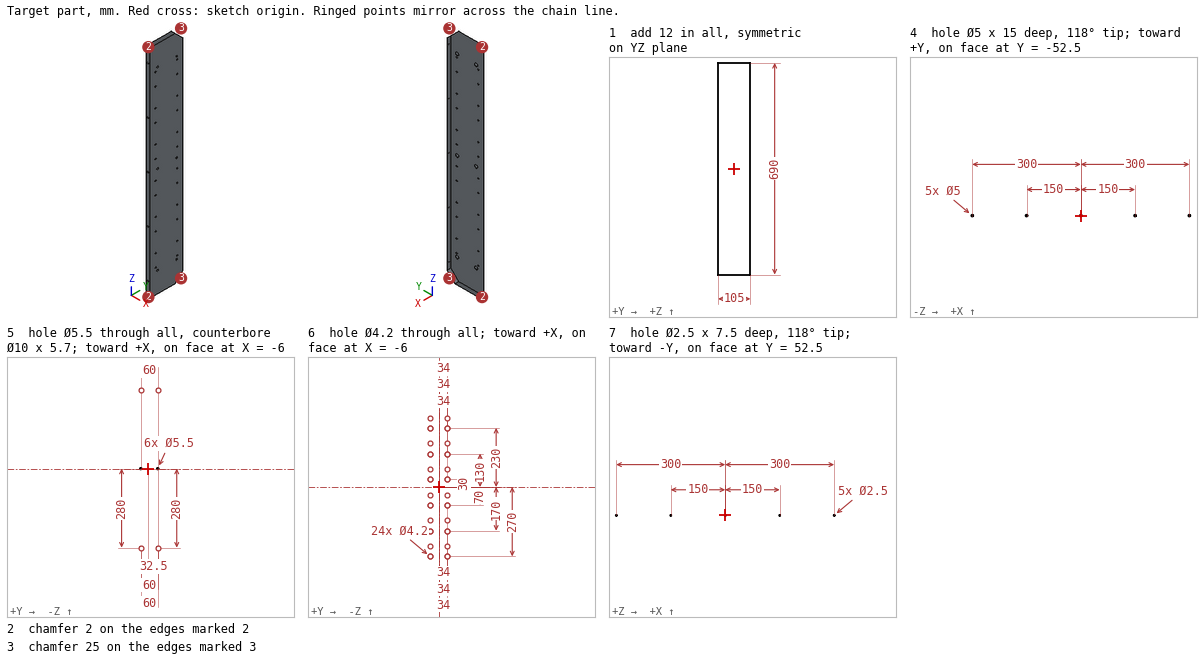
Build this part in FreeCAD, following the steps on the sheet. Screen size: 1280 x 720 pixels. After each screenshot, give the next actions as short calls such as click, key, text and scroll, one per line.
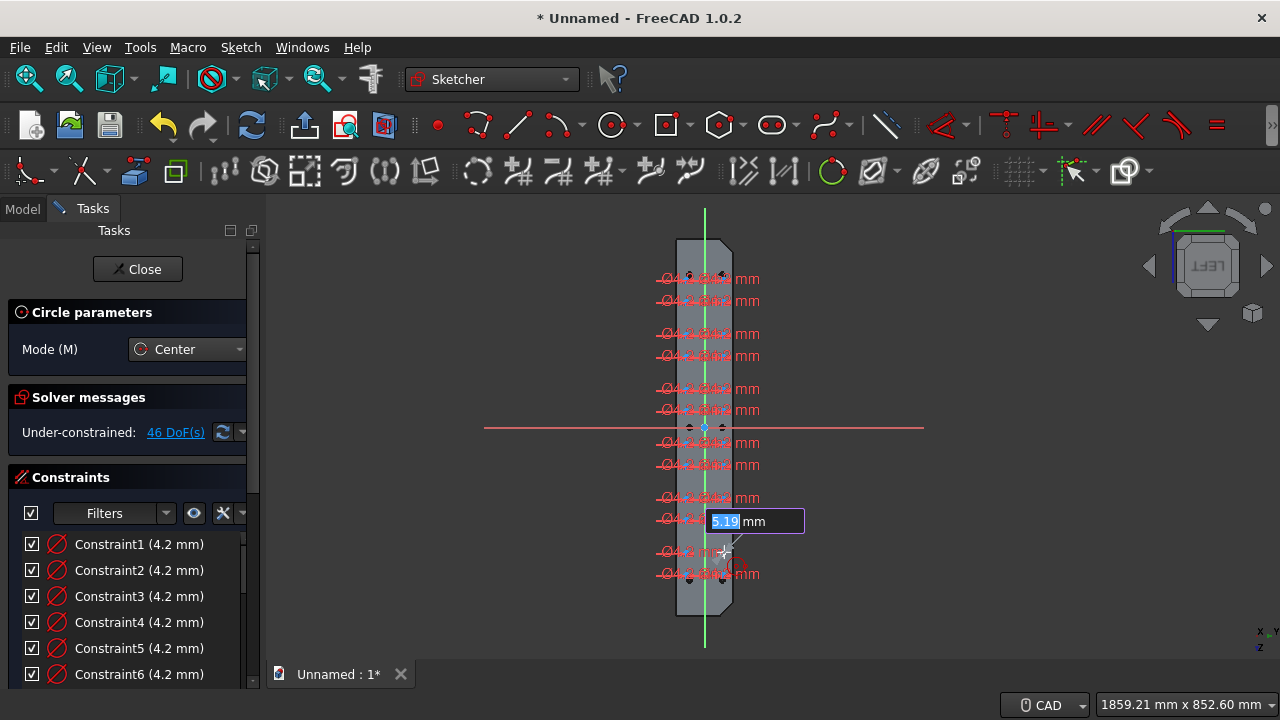
text(4.2)
key(Return)
key(Escape)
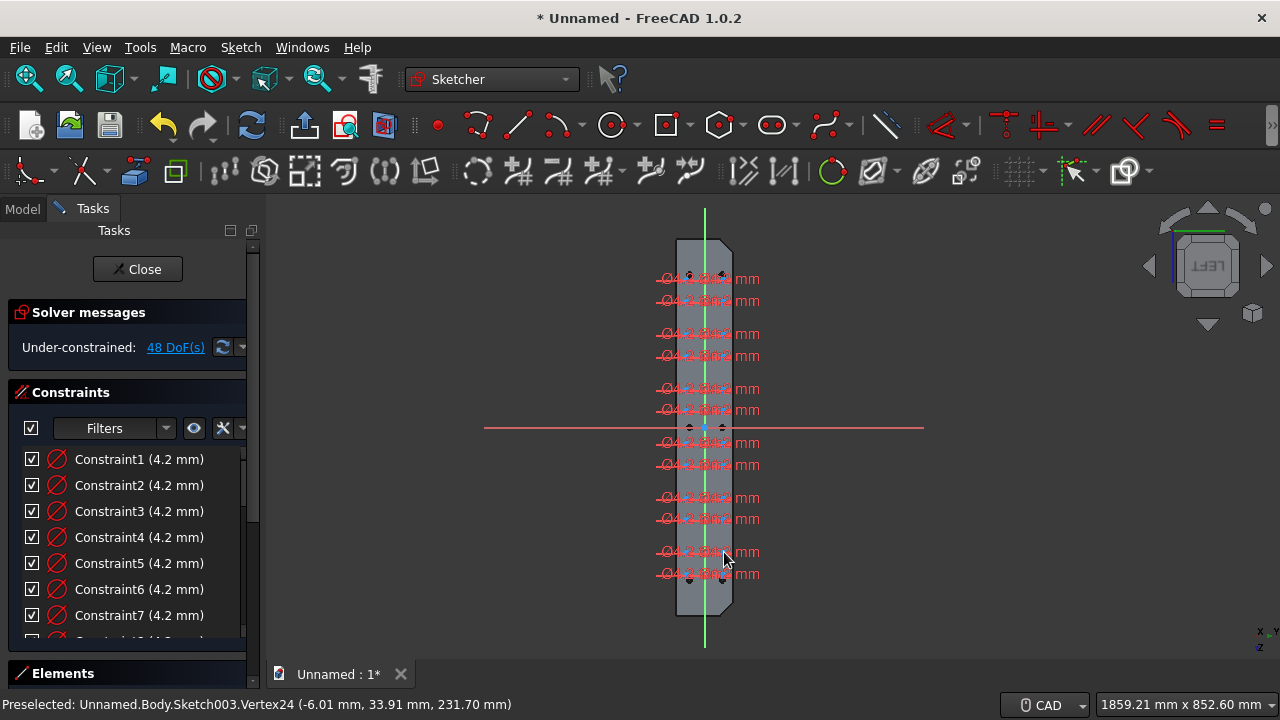
click(723, 576)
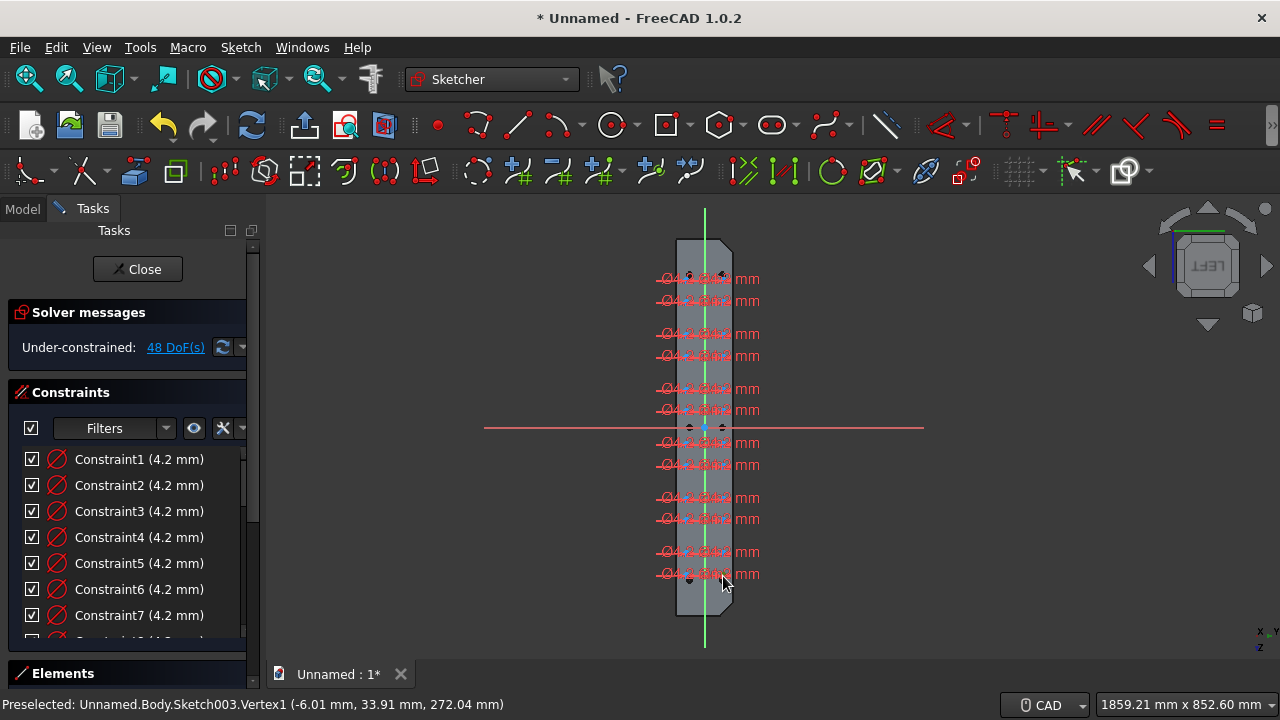
click(686, 576)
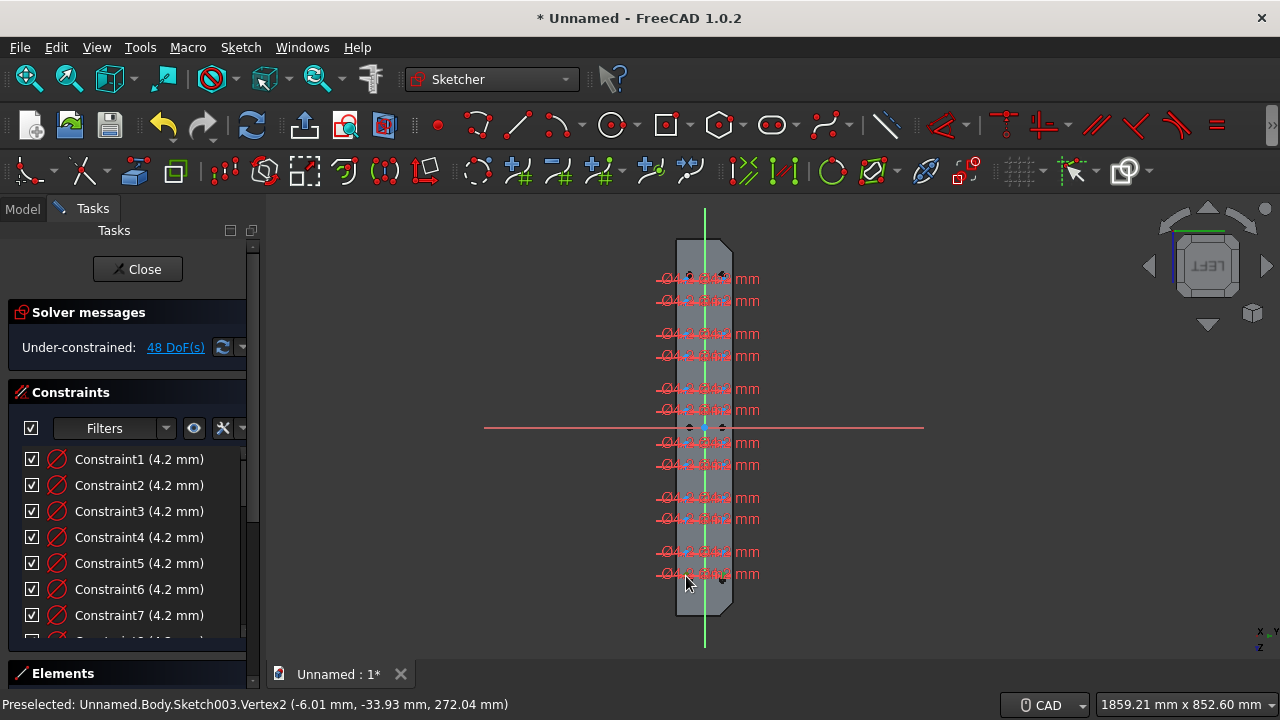
click(705, 602)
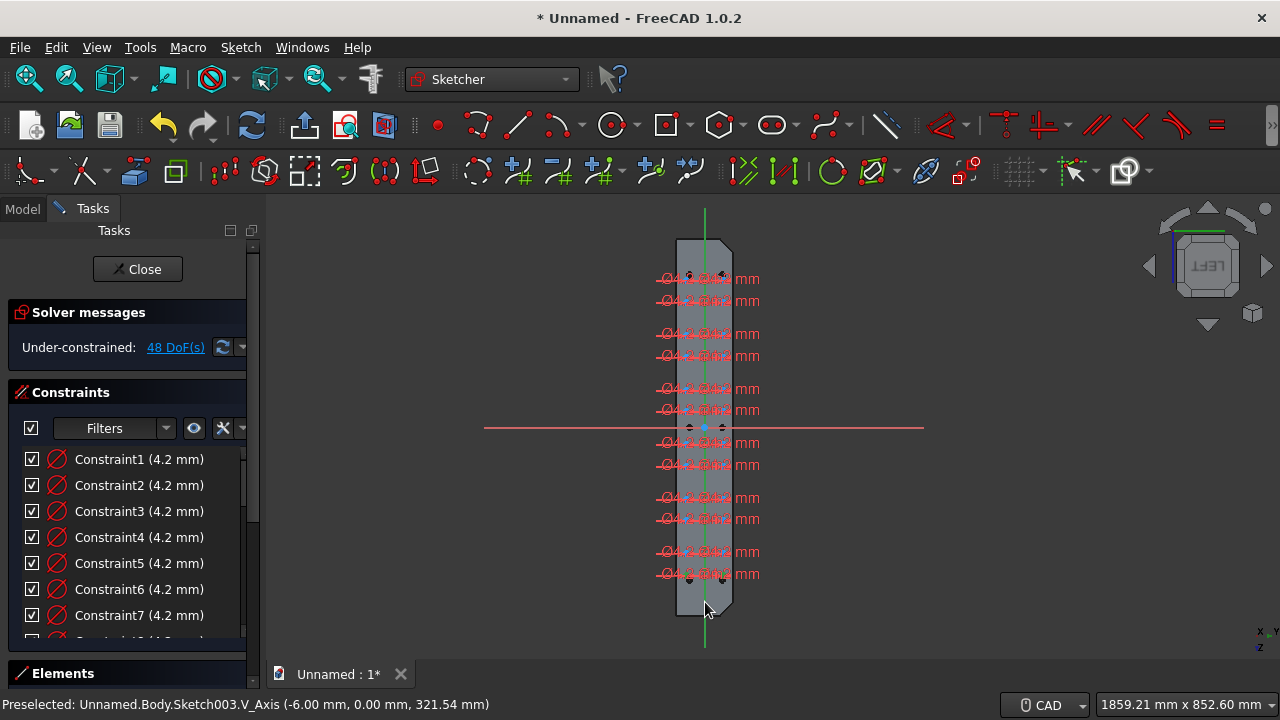
key(s)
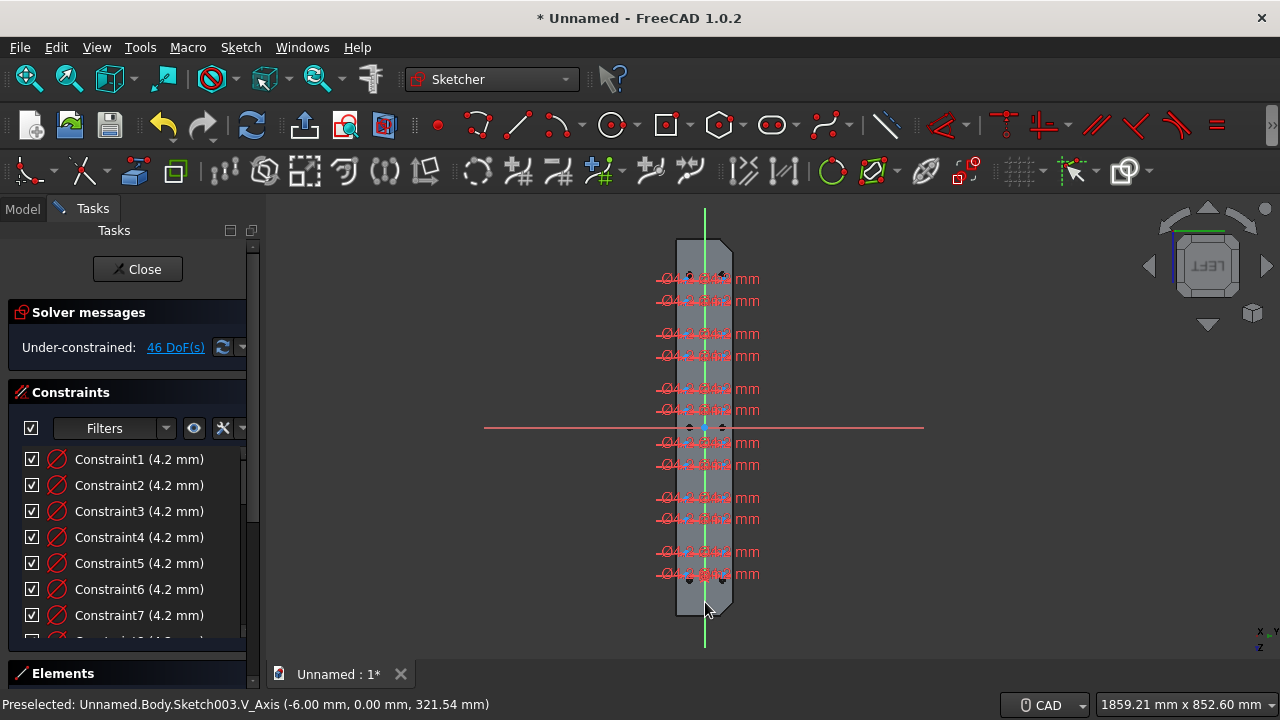
click(723, 521)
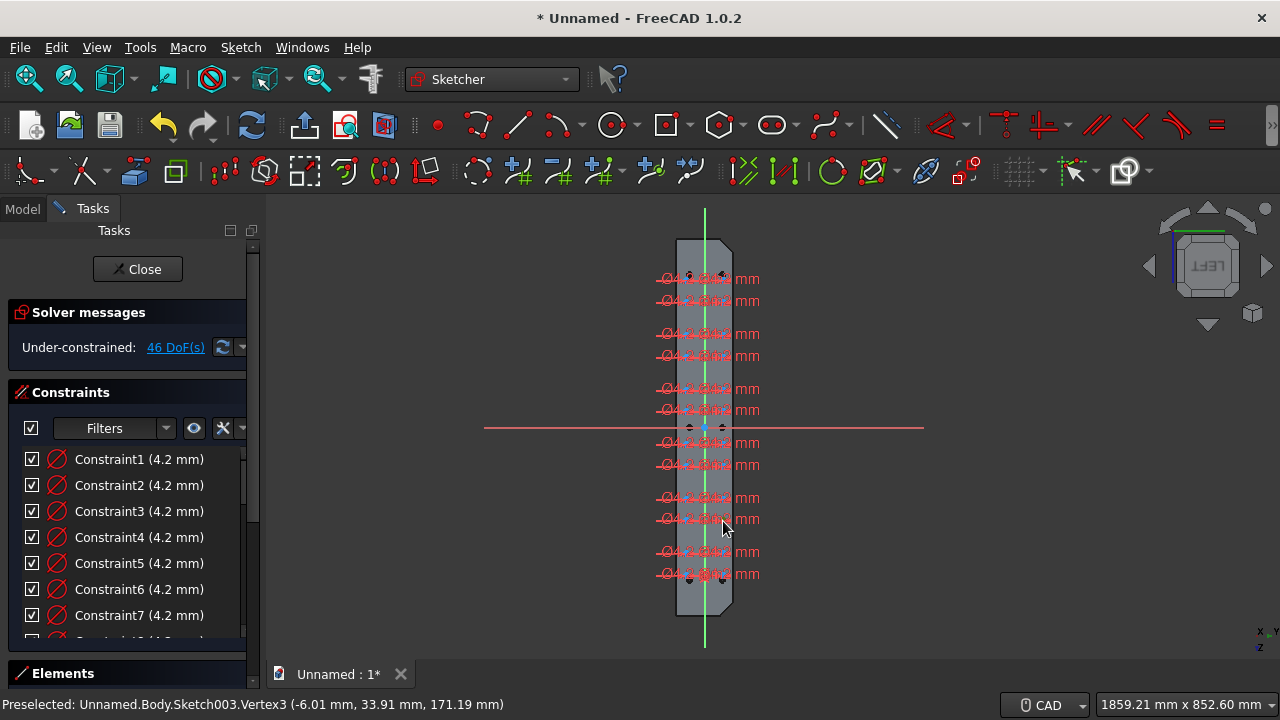
click(686, 521)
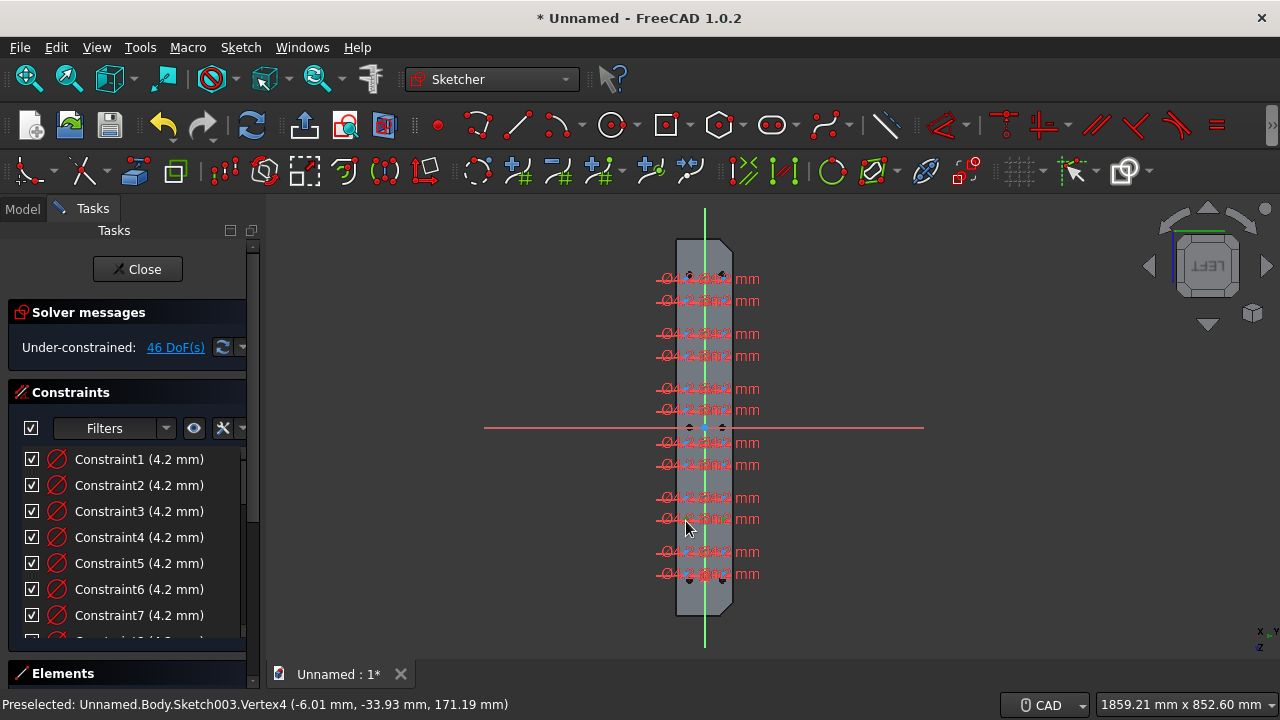
click(705, 602)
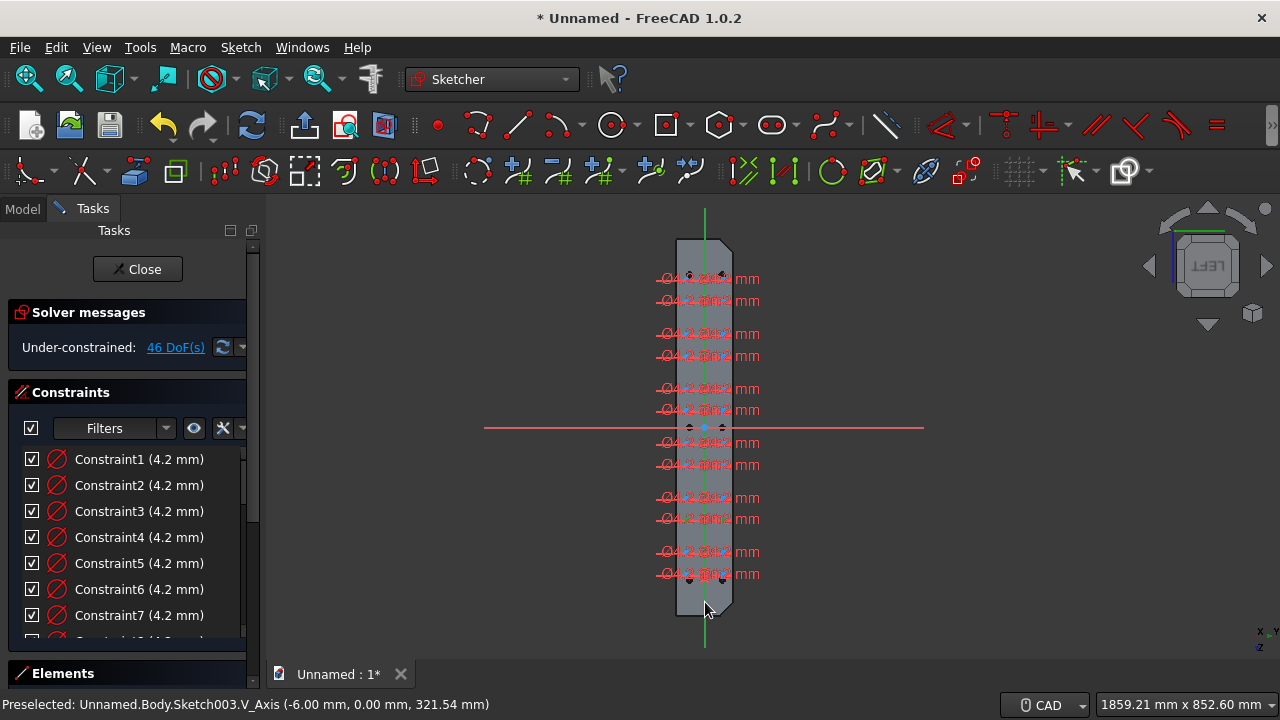
key(s)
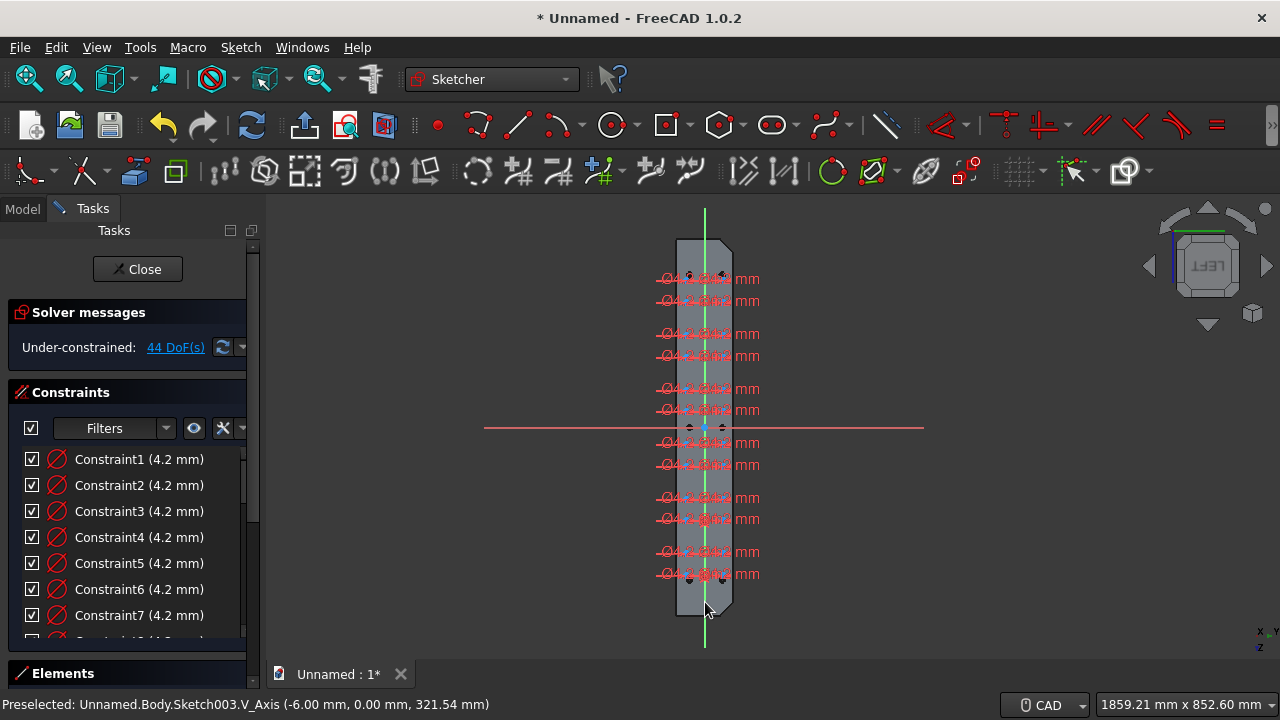
click(723, 467)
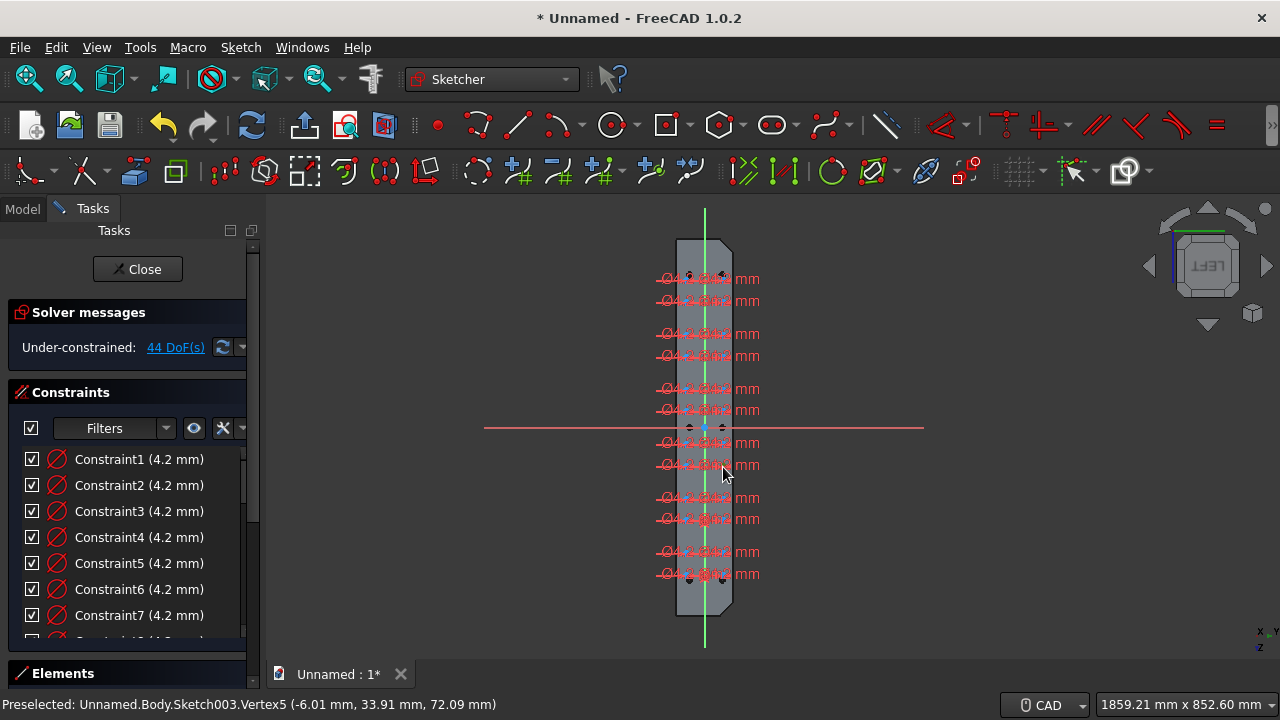
click(686, 467)